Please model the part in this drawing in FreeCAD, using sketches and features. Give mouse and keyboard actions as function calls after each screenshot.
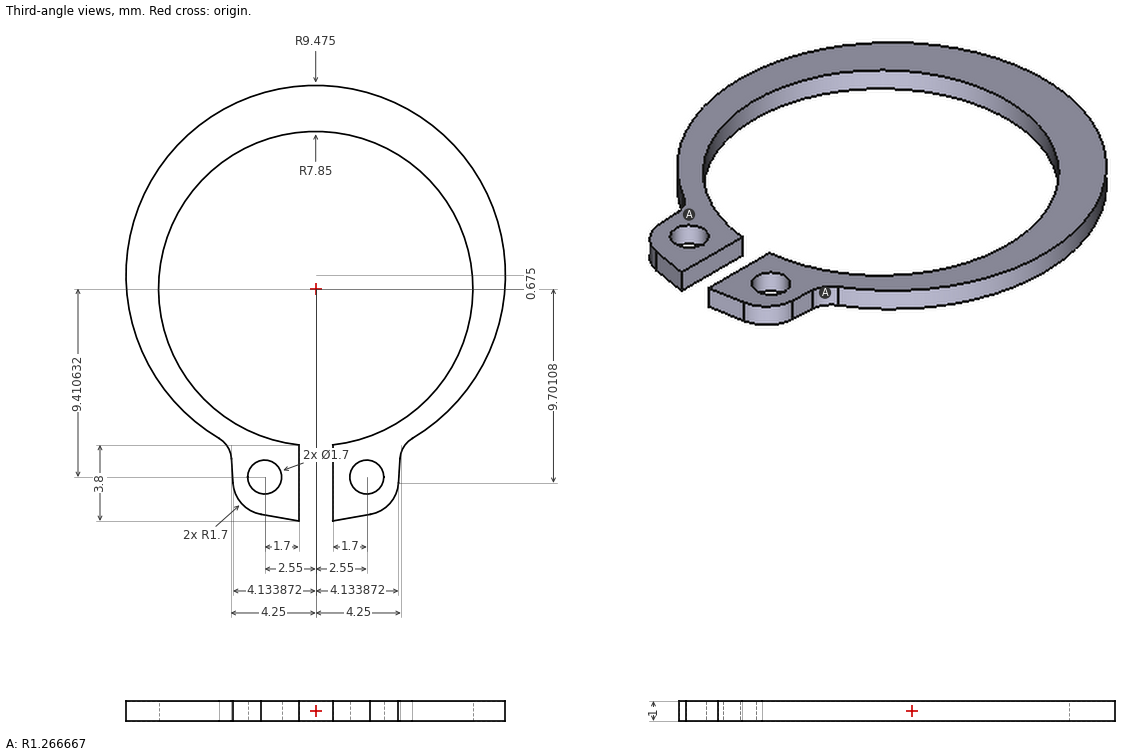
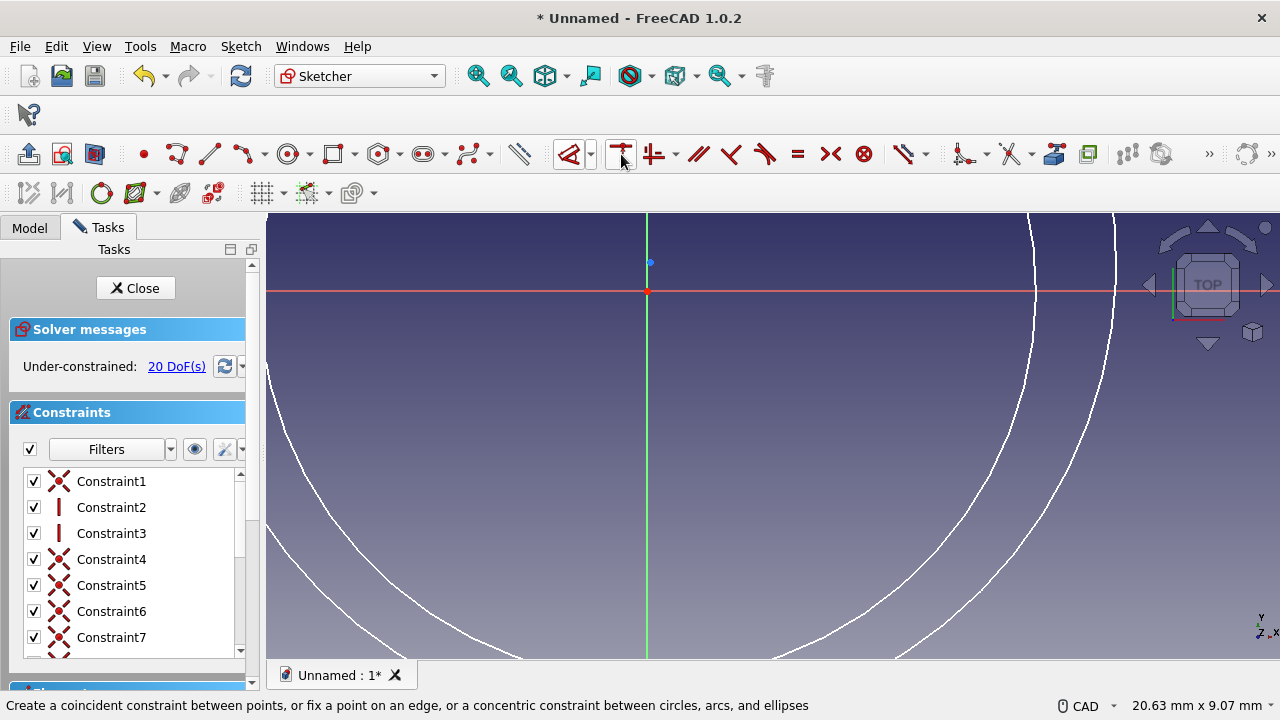
scroll(723, 472, down, 7)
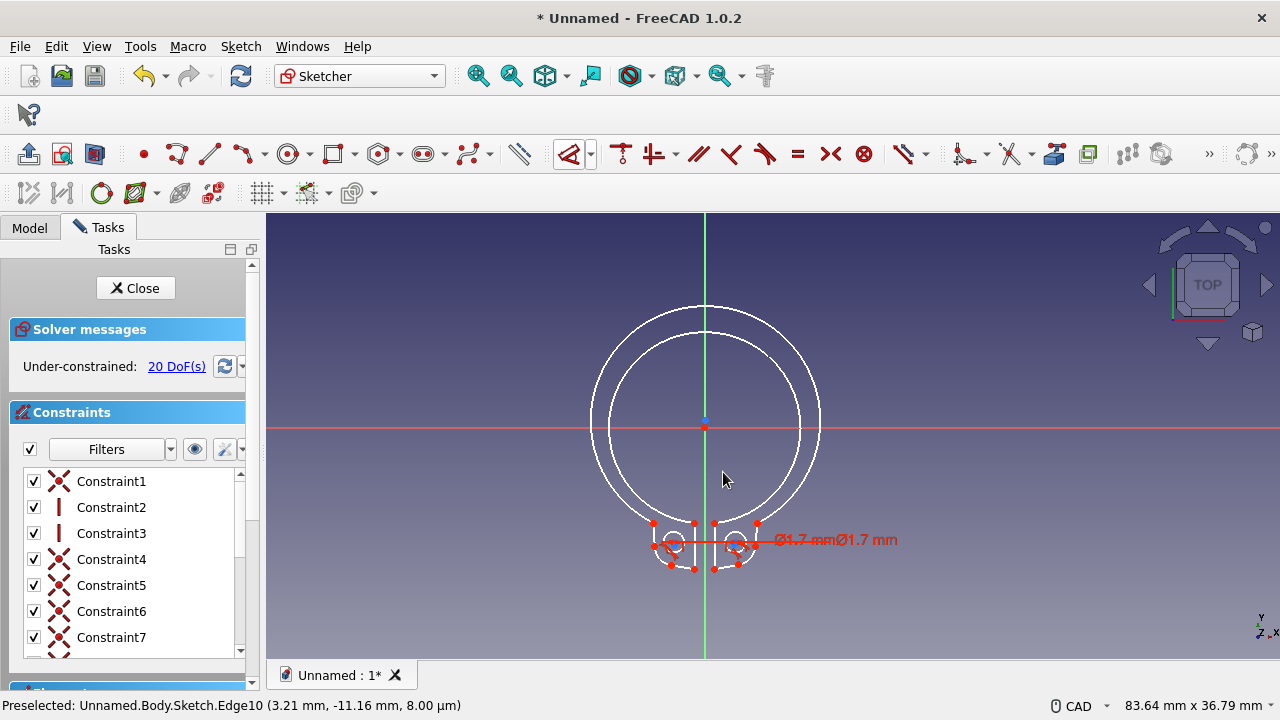
scroll(657, 555, up, 3)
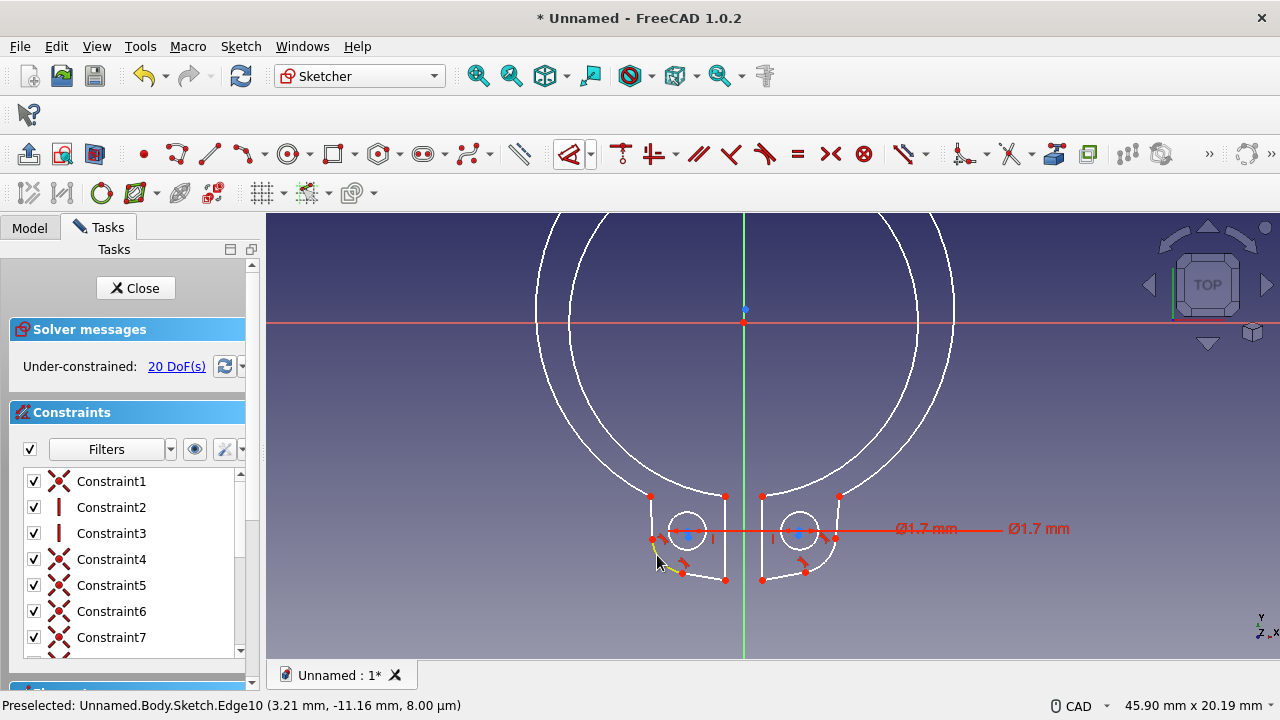
click(656, 553)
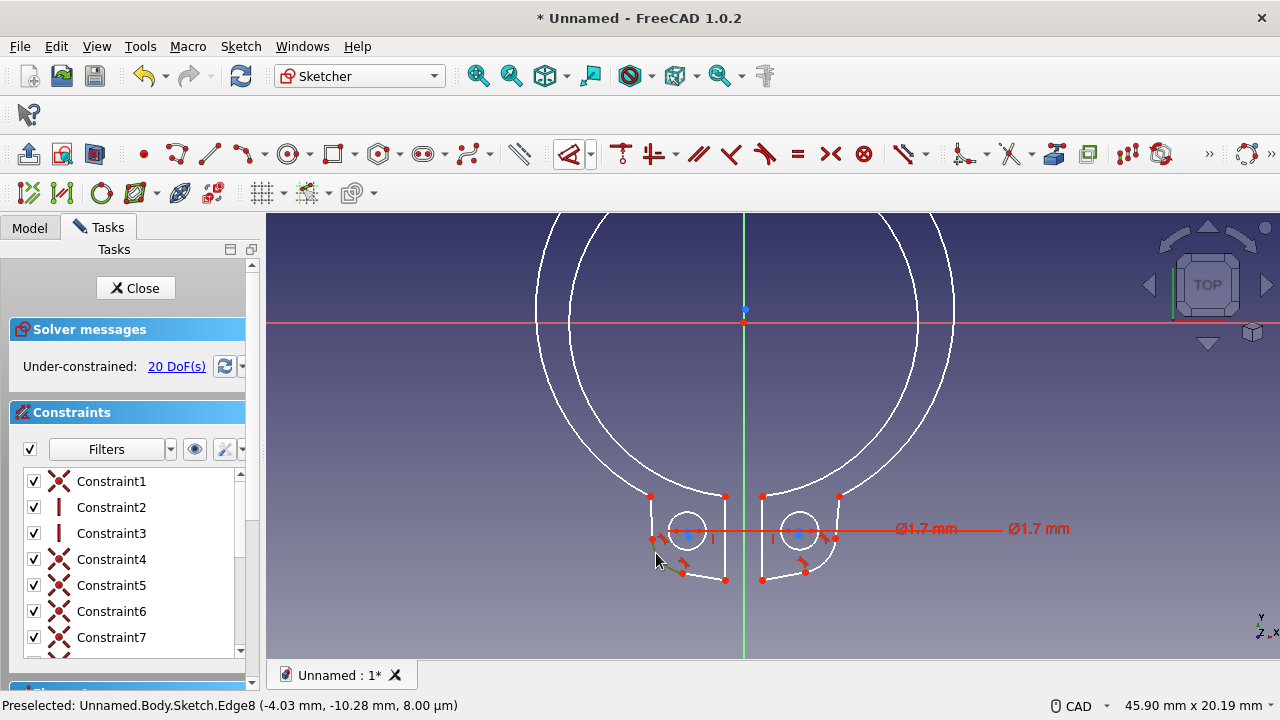
click(819, 567)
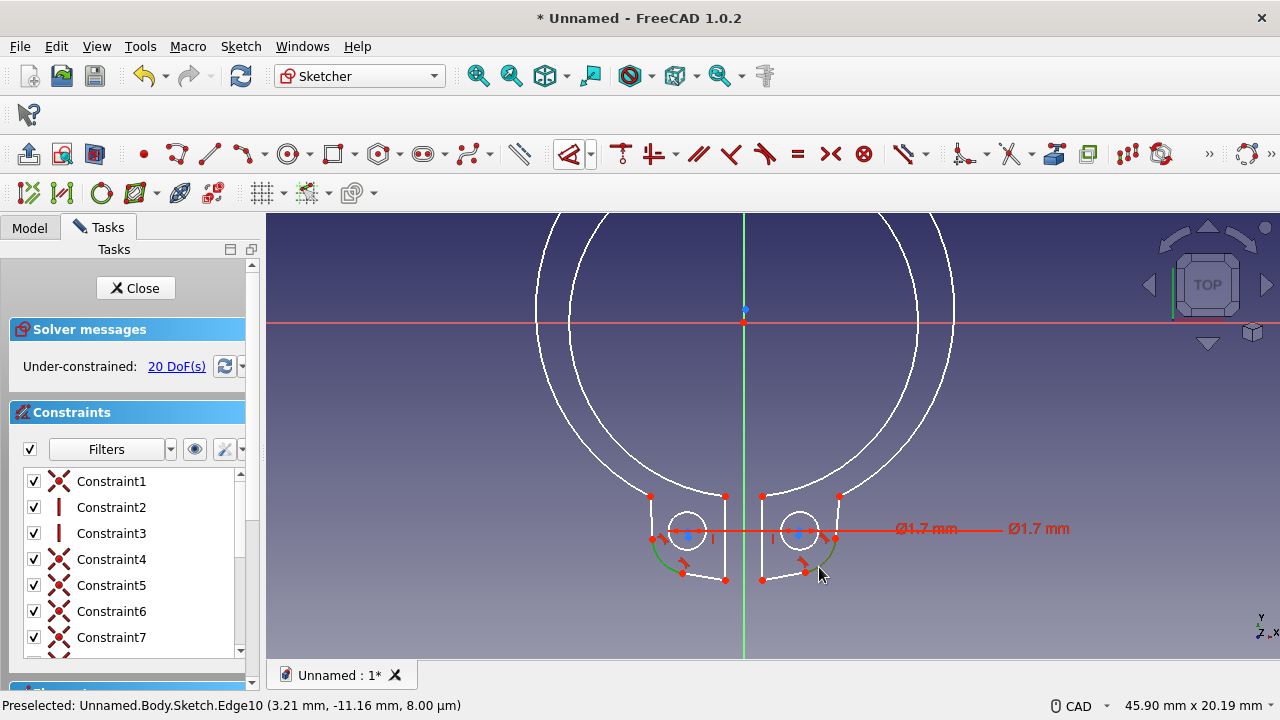
click(798, 154)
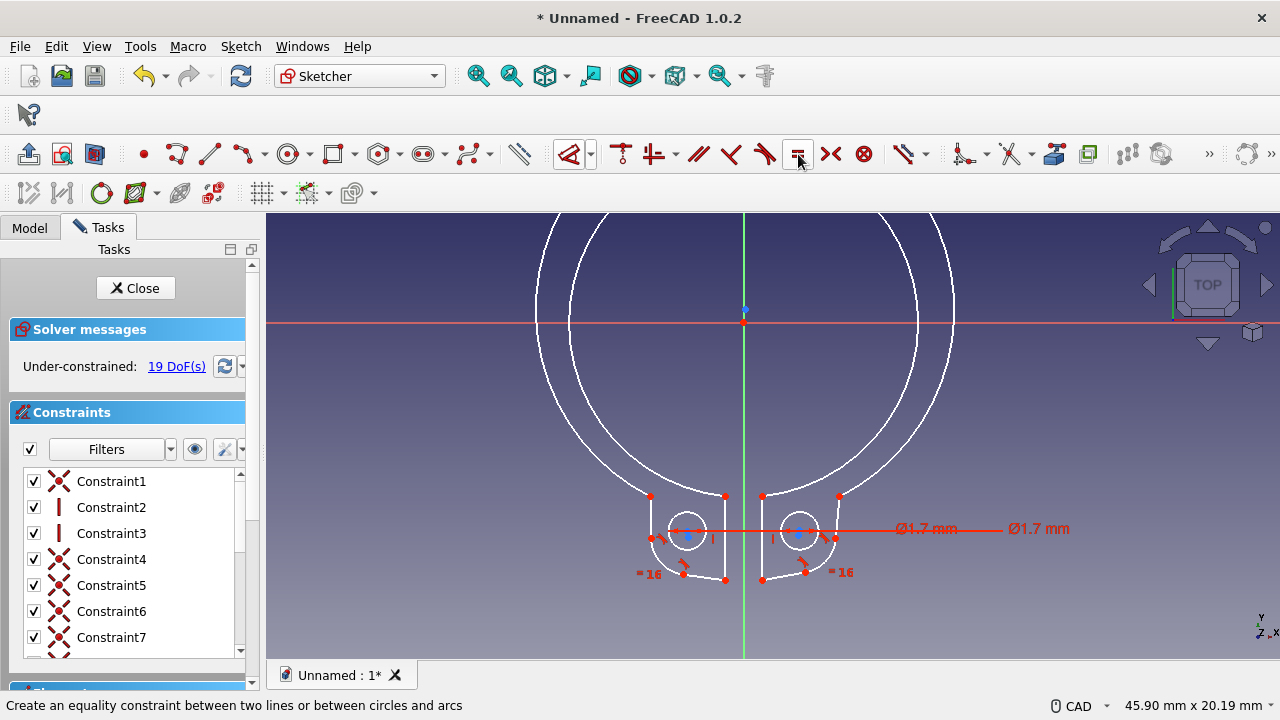
click(745, 310)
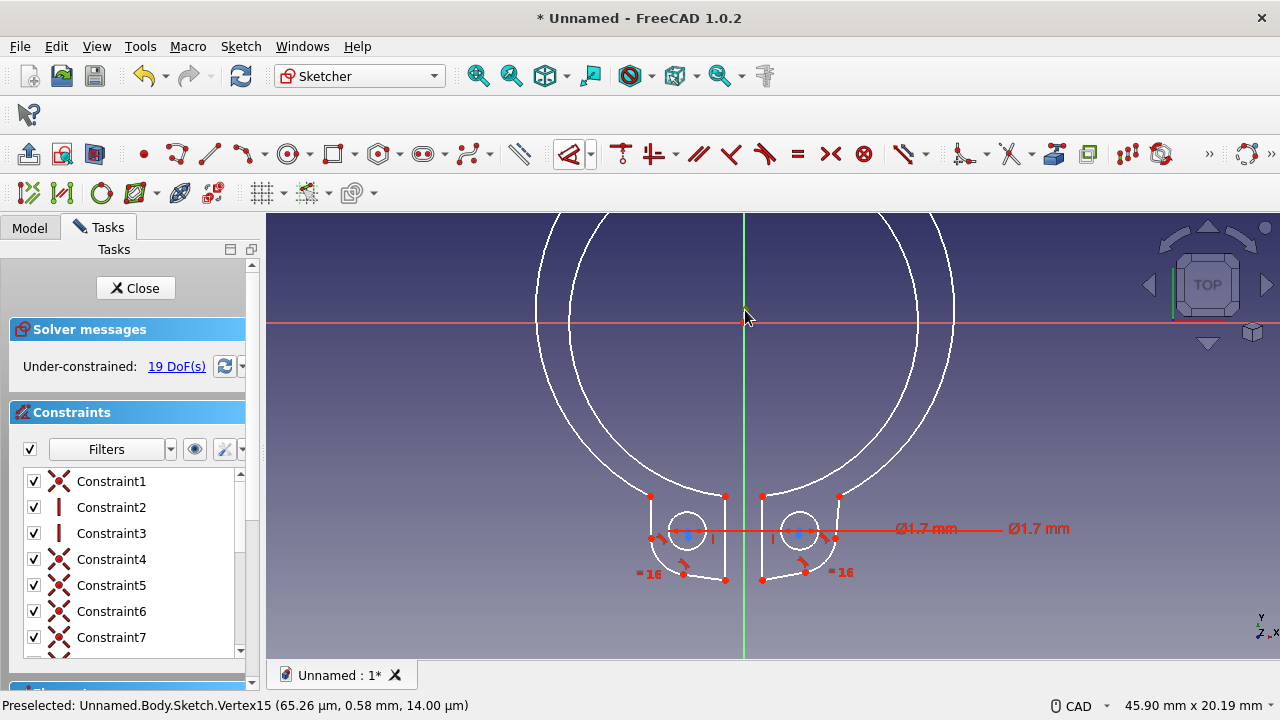
click(744, 464)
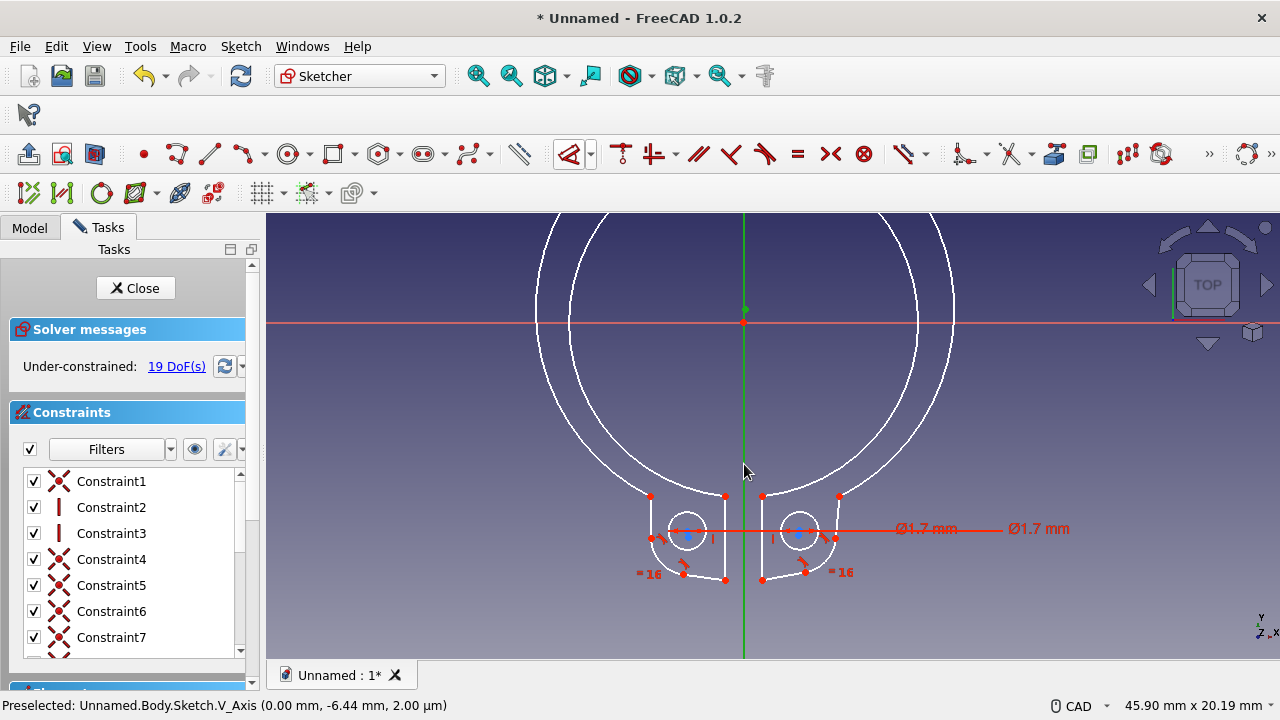
click(621, 154)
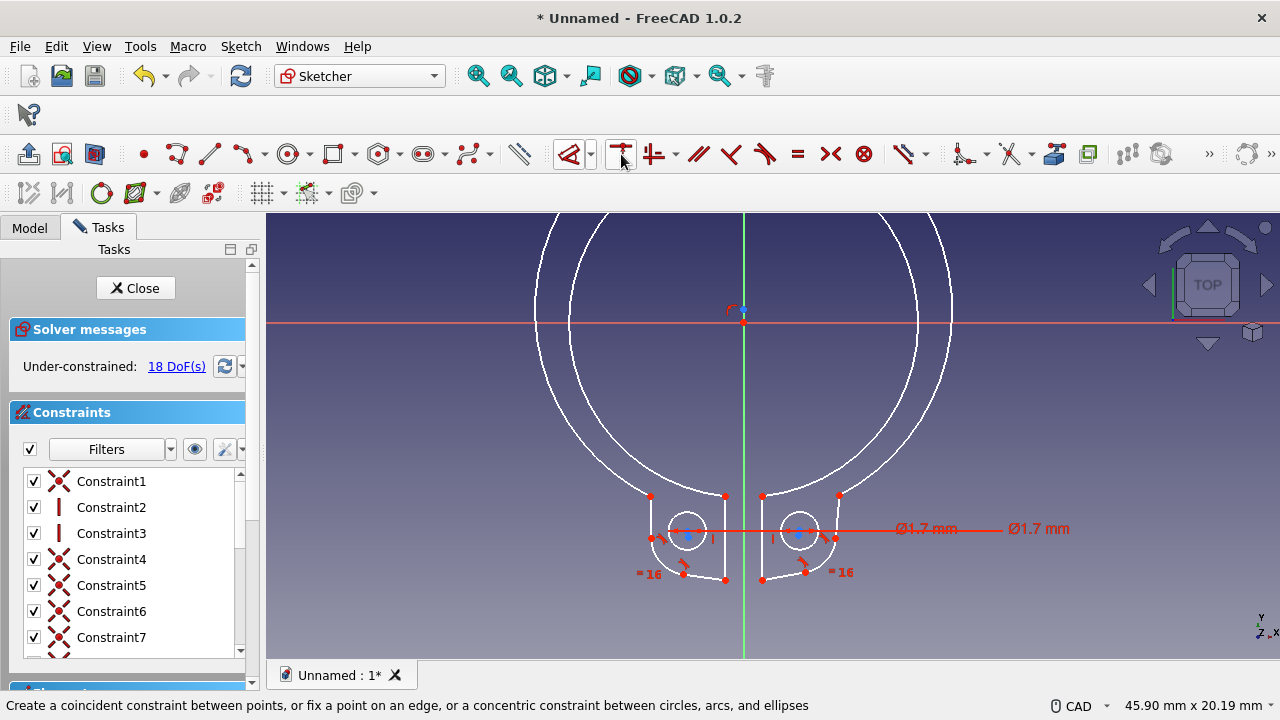
scroll(657, 554, down, 3)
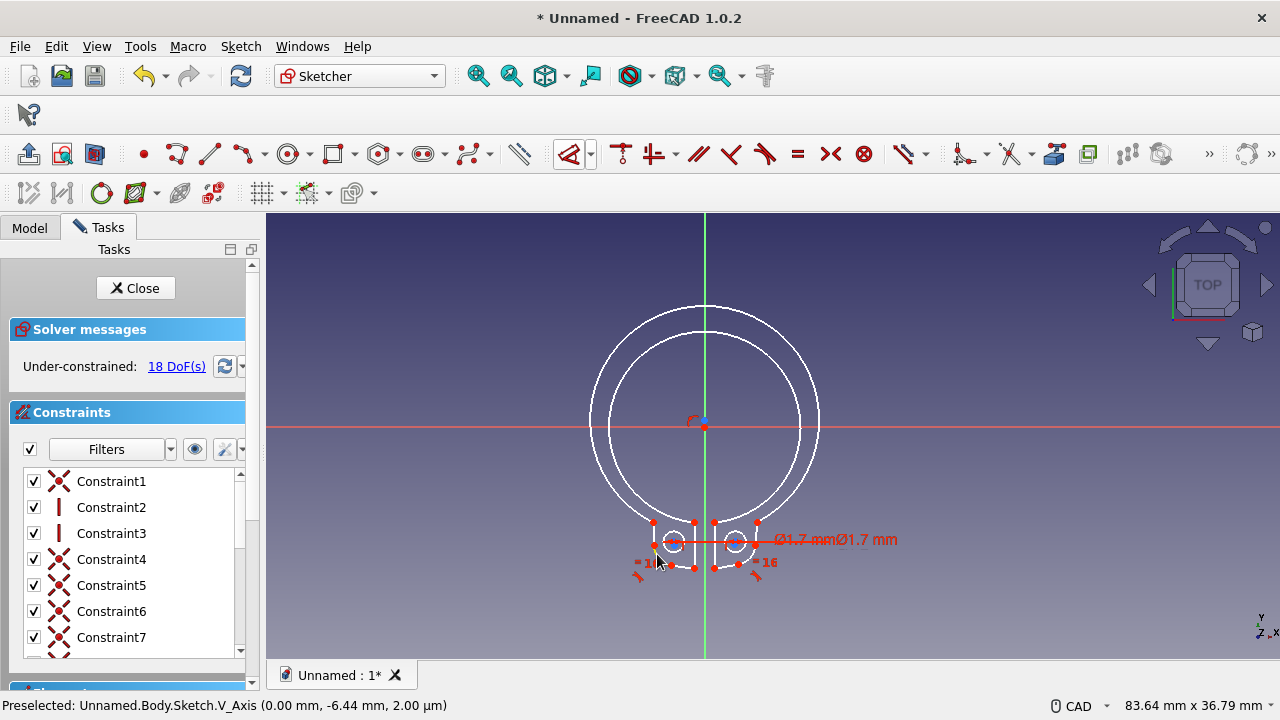
click(805, 365)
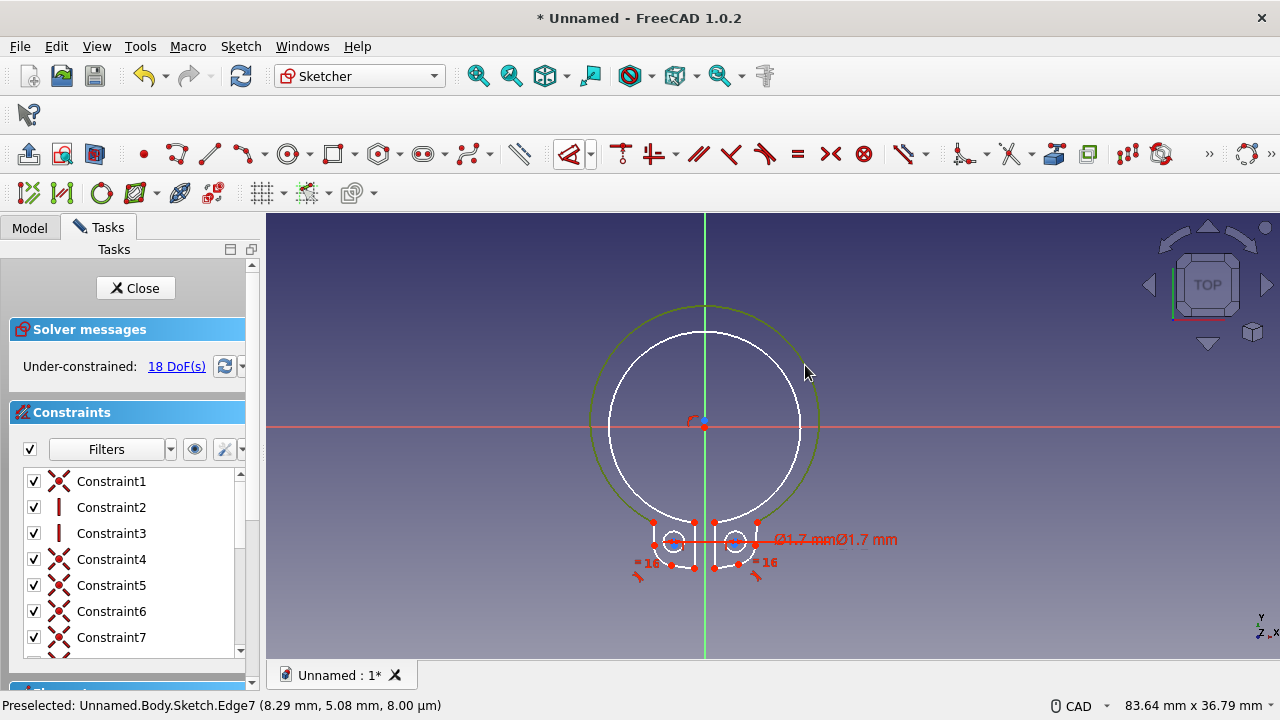
click(590, 154)